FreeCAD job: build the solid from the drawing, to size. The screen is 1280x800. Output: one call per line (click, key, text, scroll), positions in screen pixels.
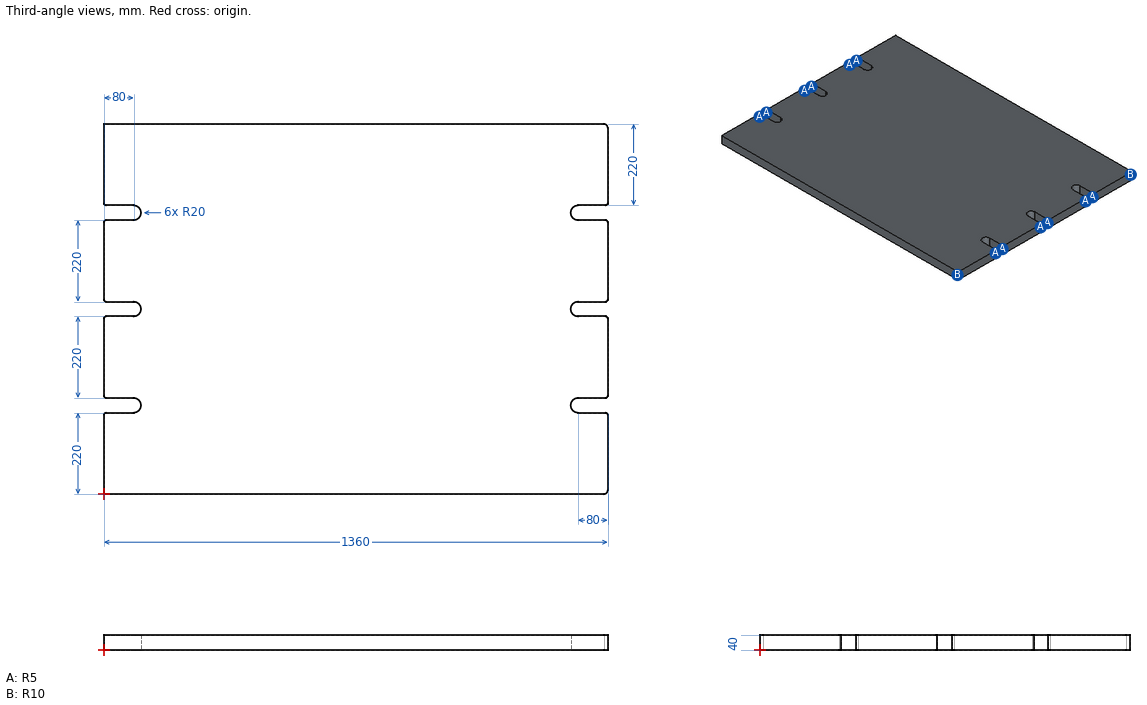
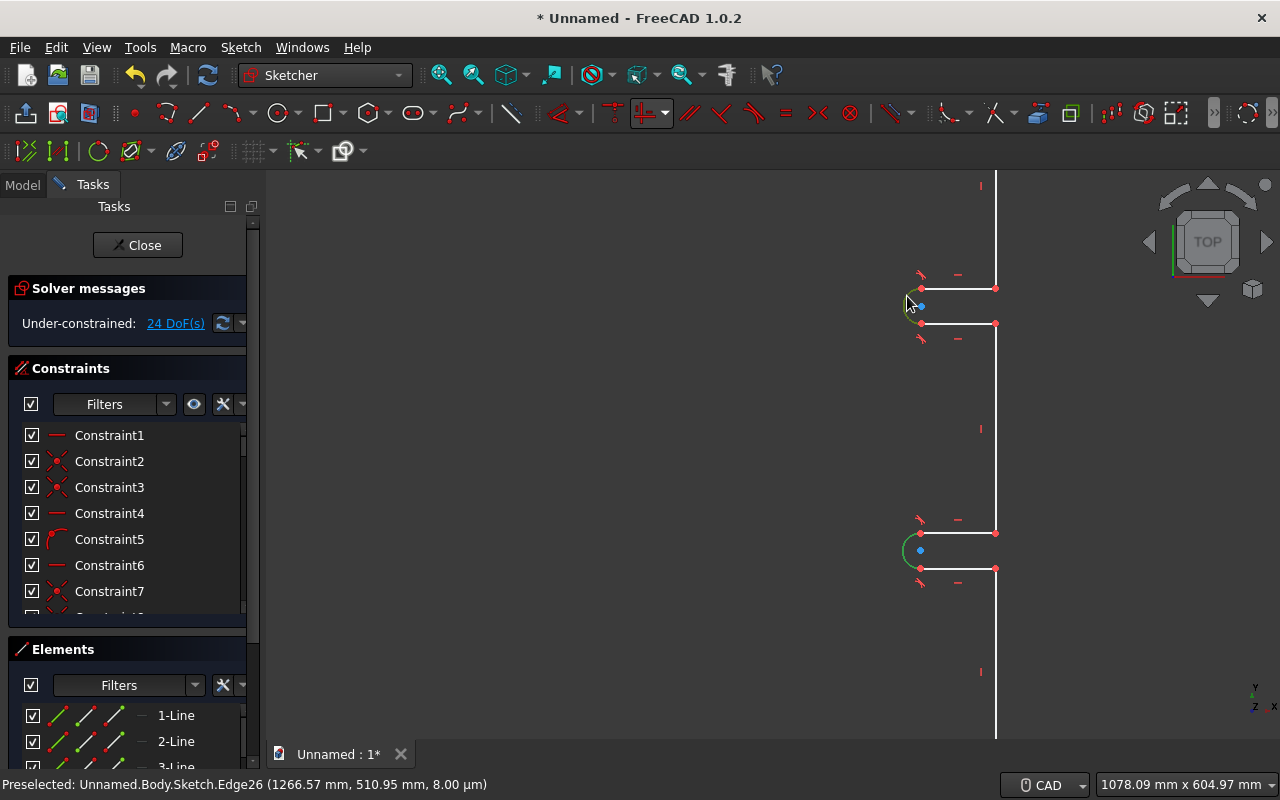
scroll(907, 542, down, 5)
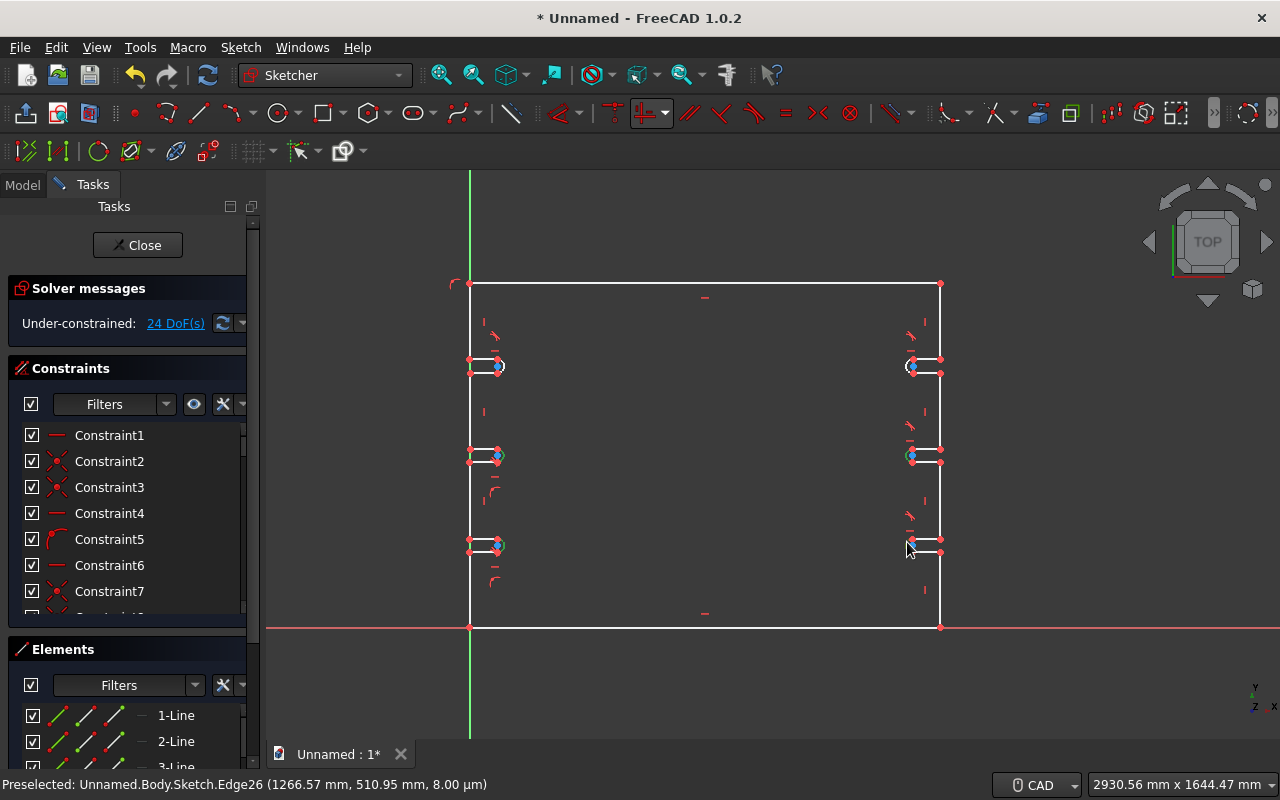
scroll(907, 362, up, 4)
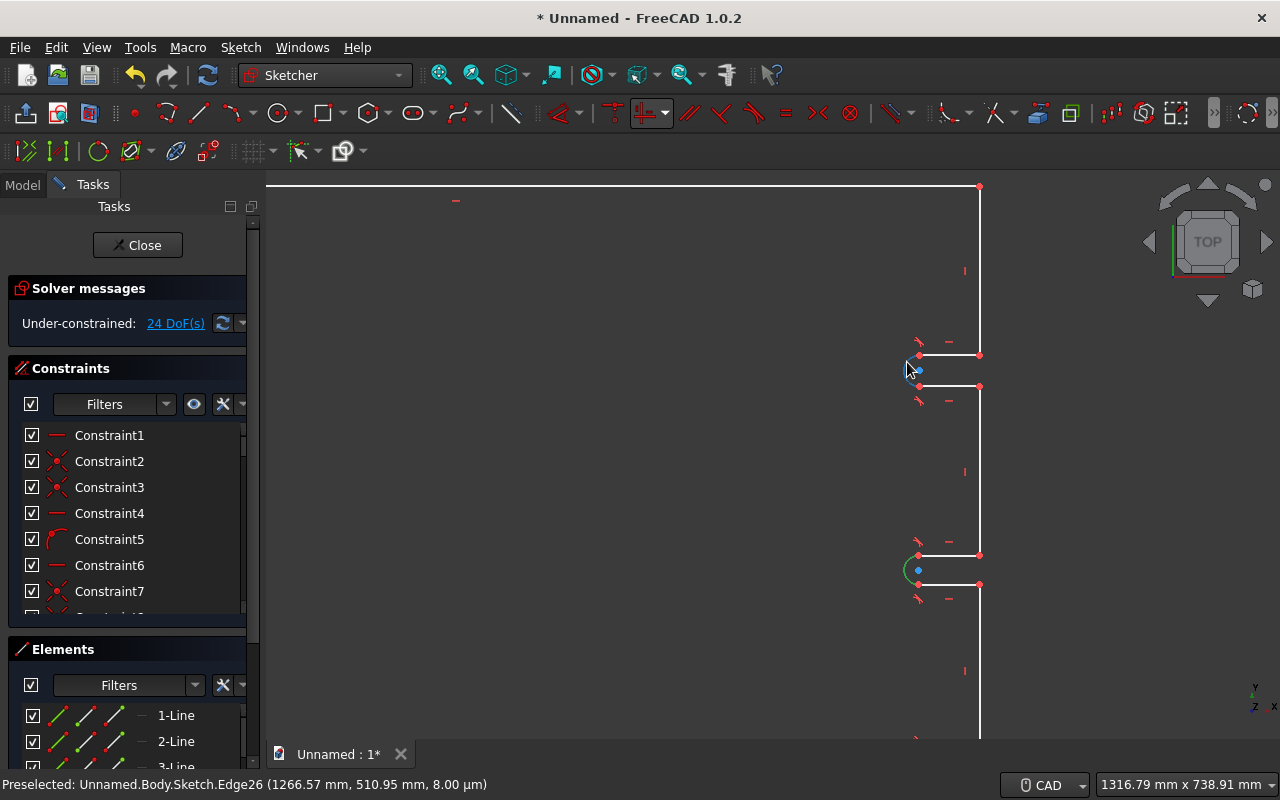
click(907, 362)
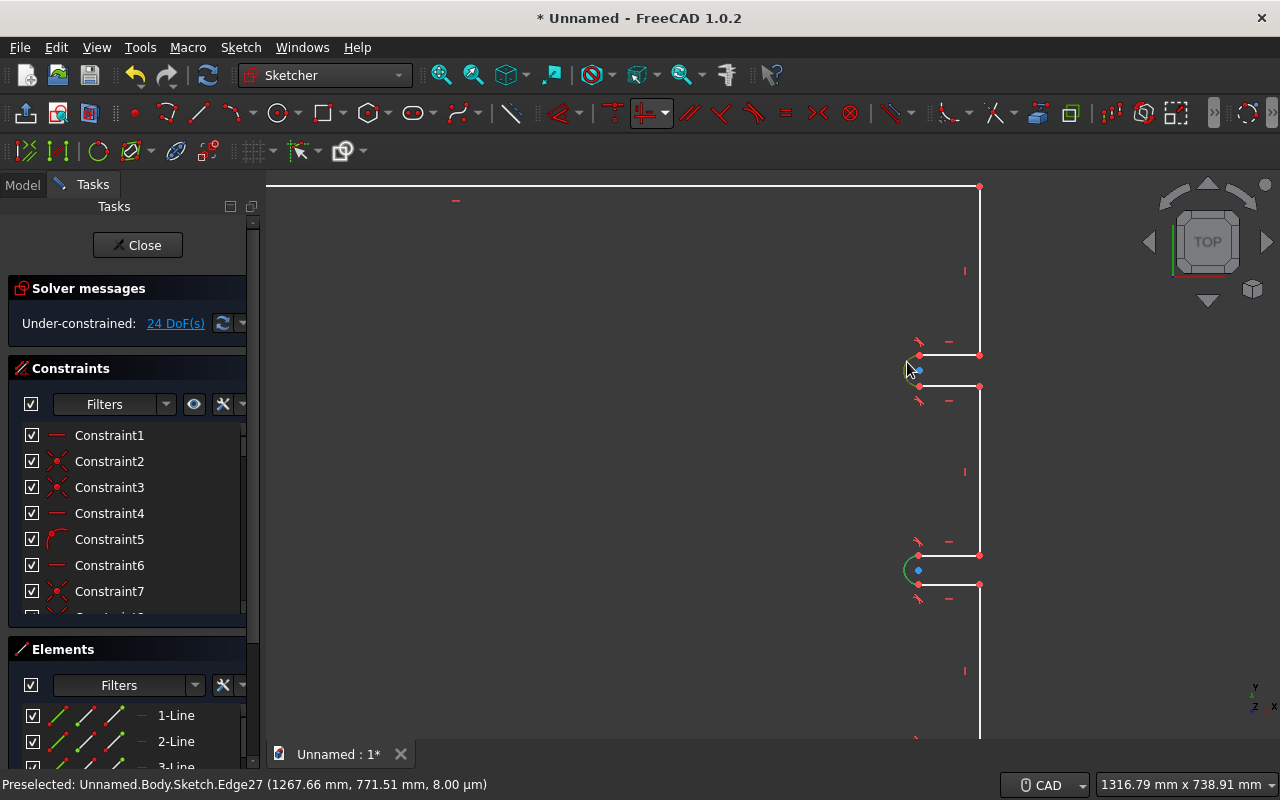
scroll(906, 362, down, 4)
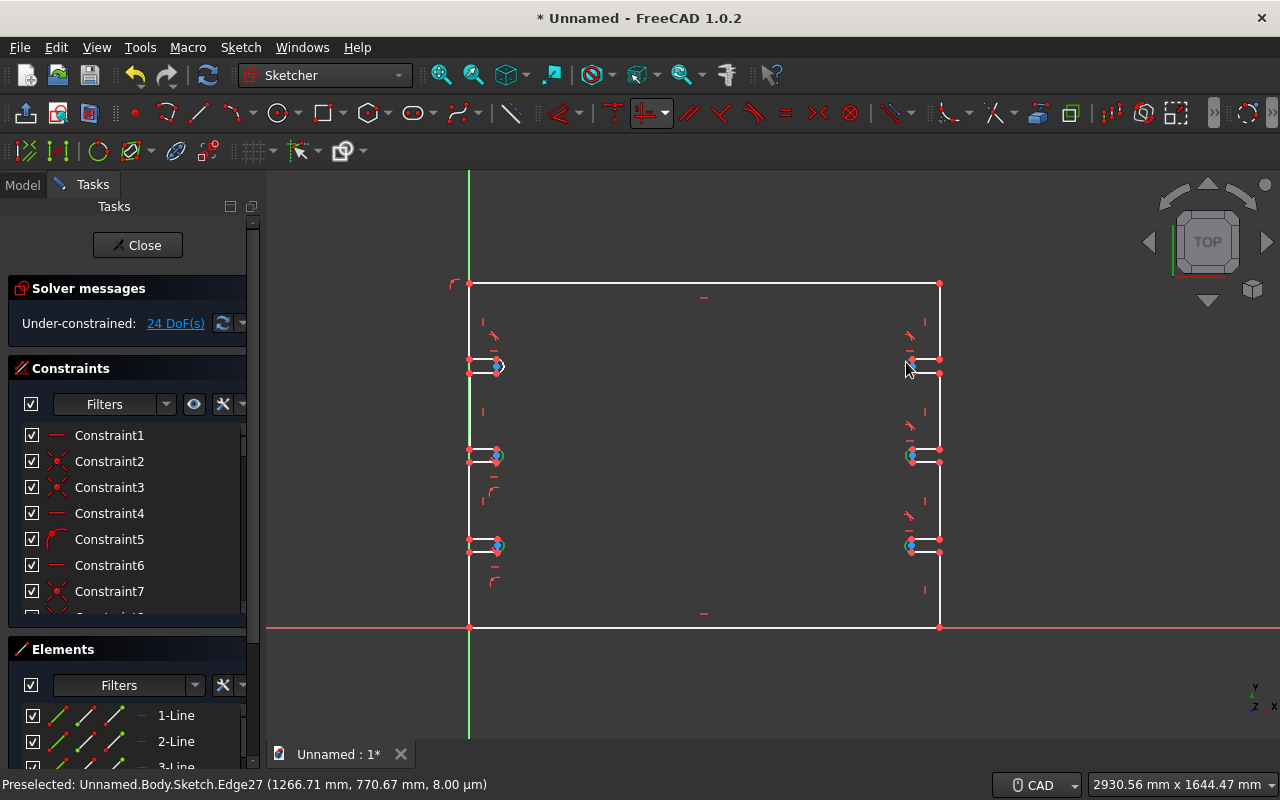
scroll(502, 370, up, 4)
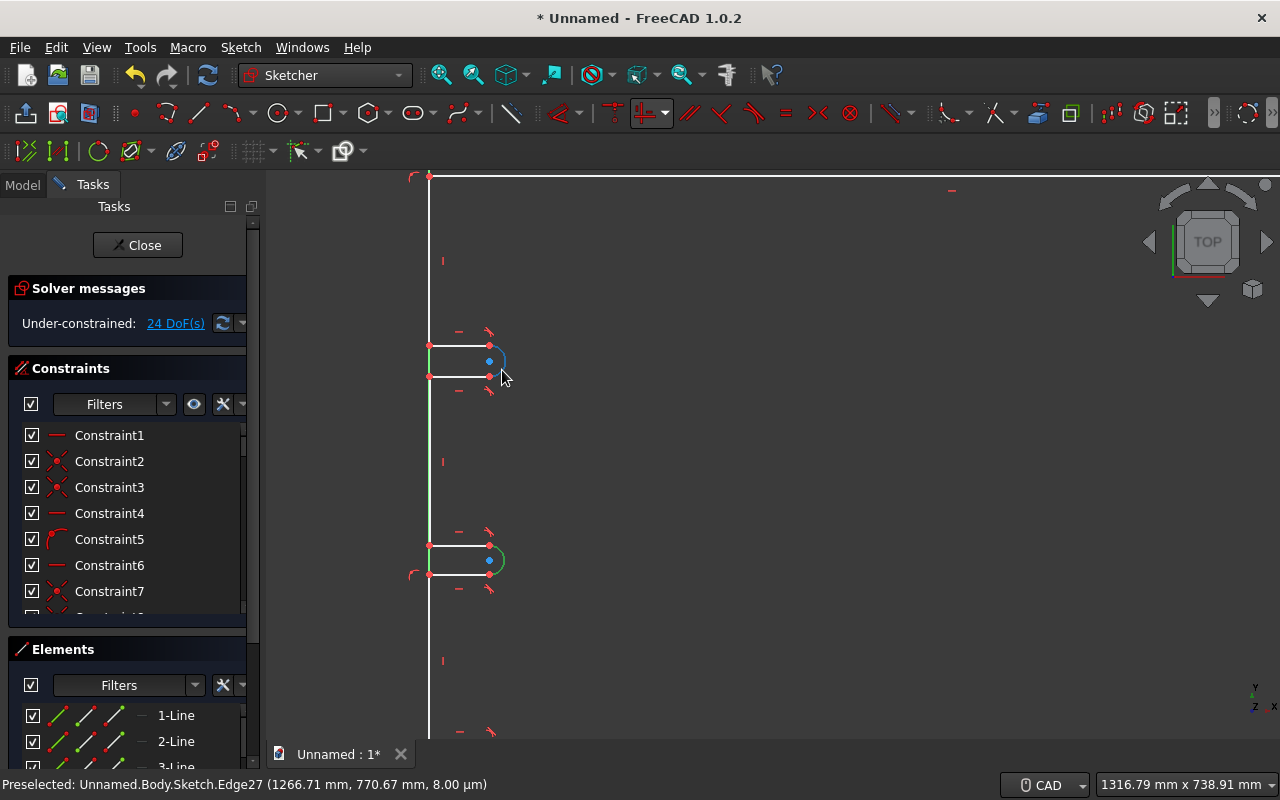
click(503, 370)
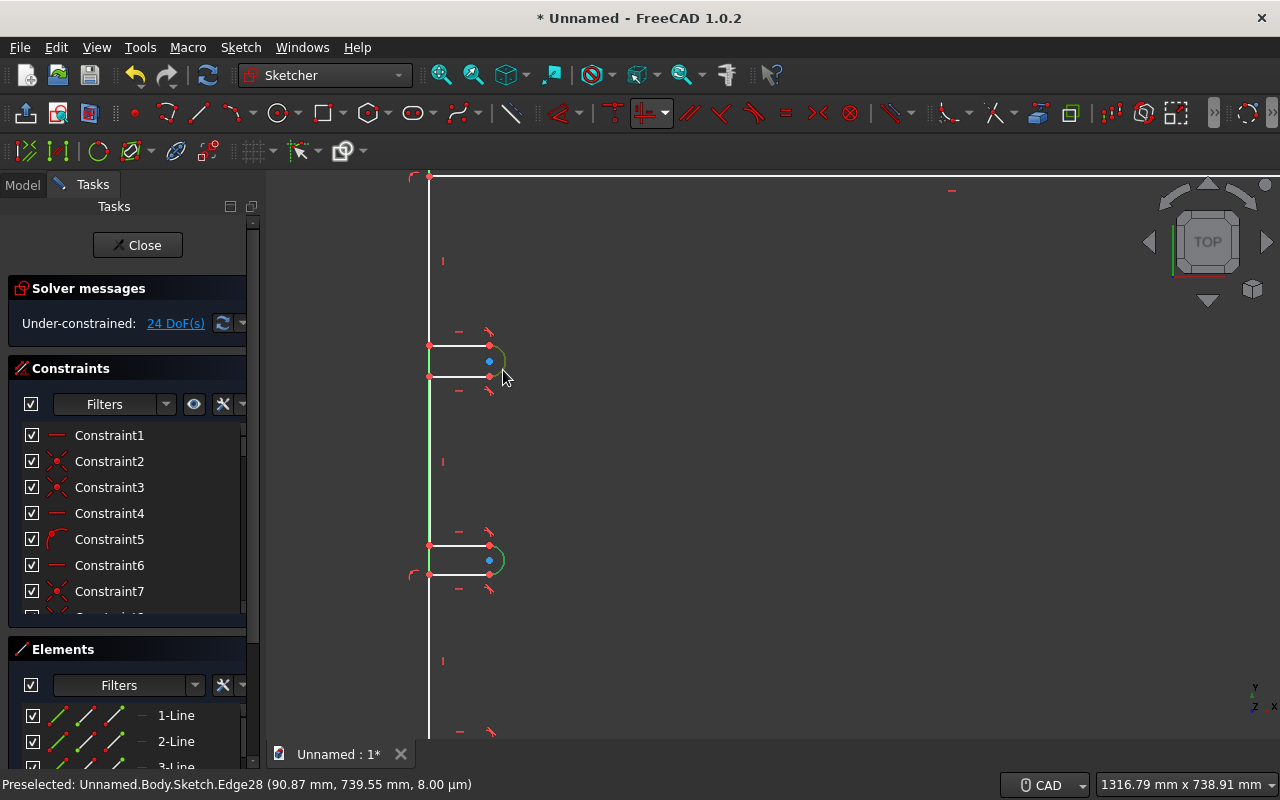
click(786, 114)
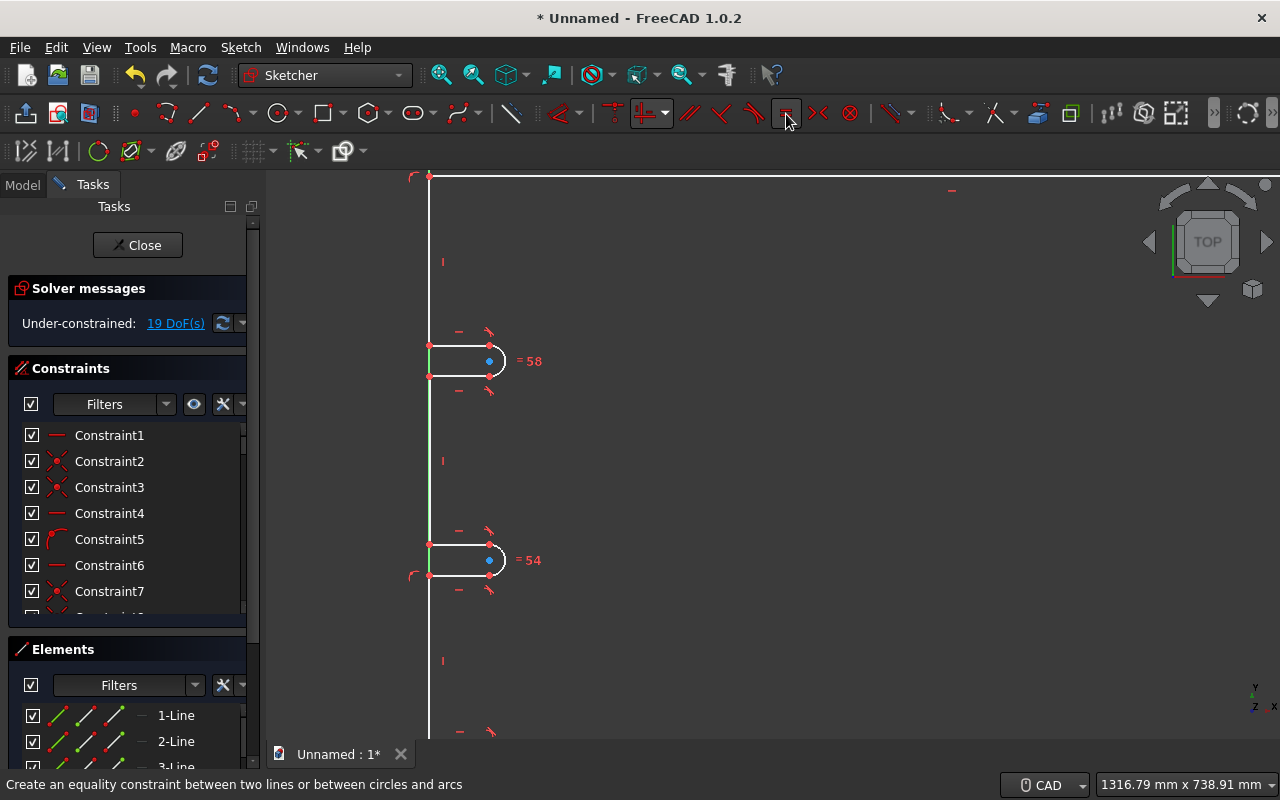
scroll(502, 569, up, 5)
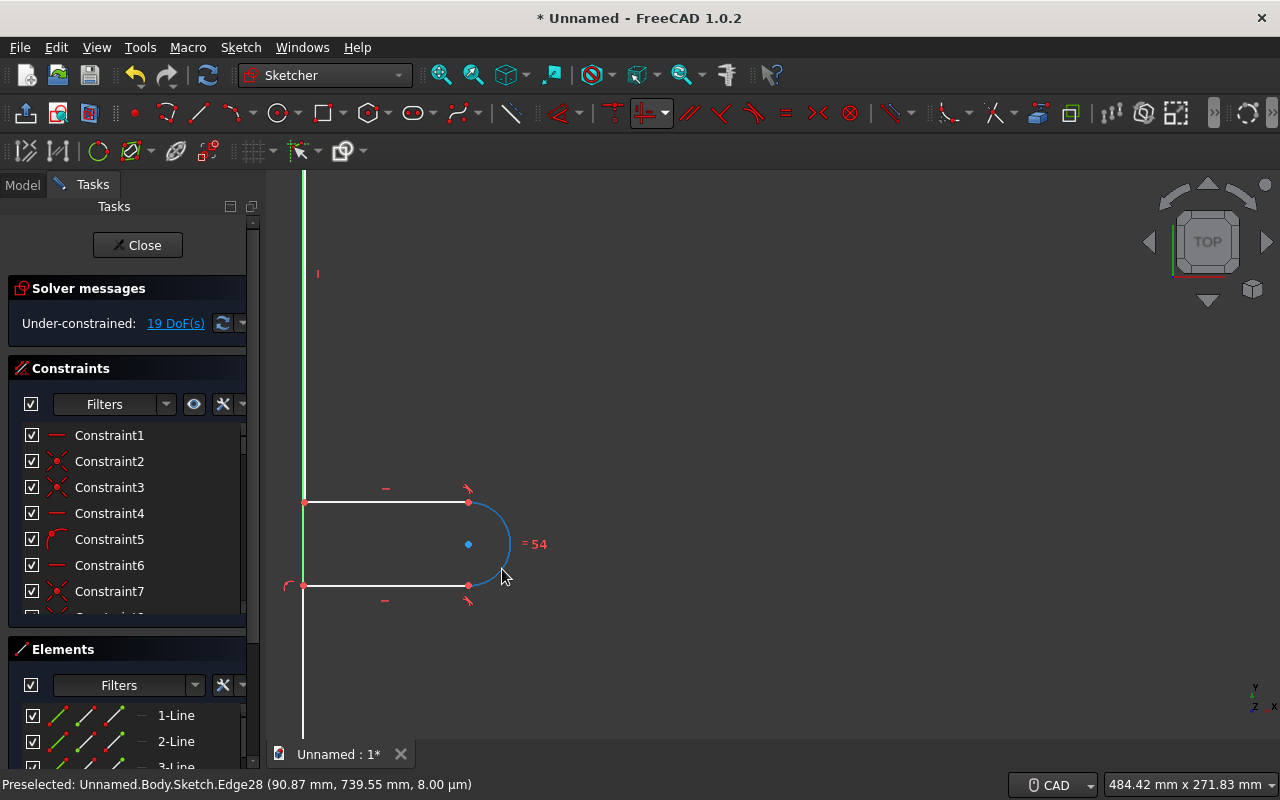
click(502, 569)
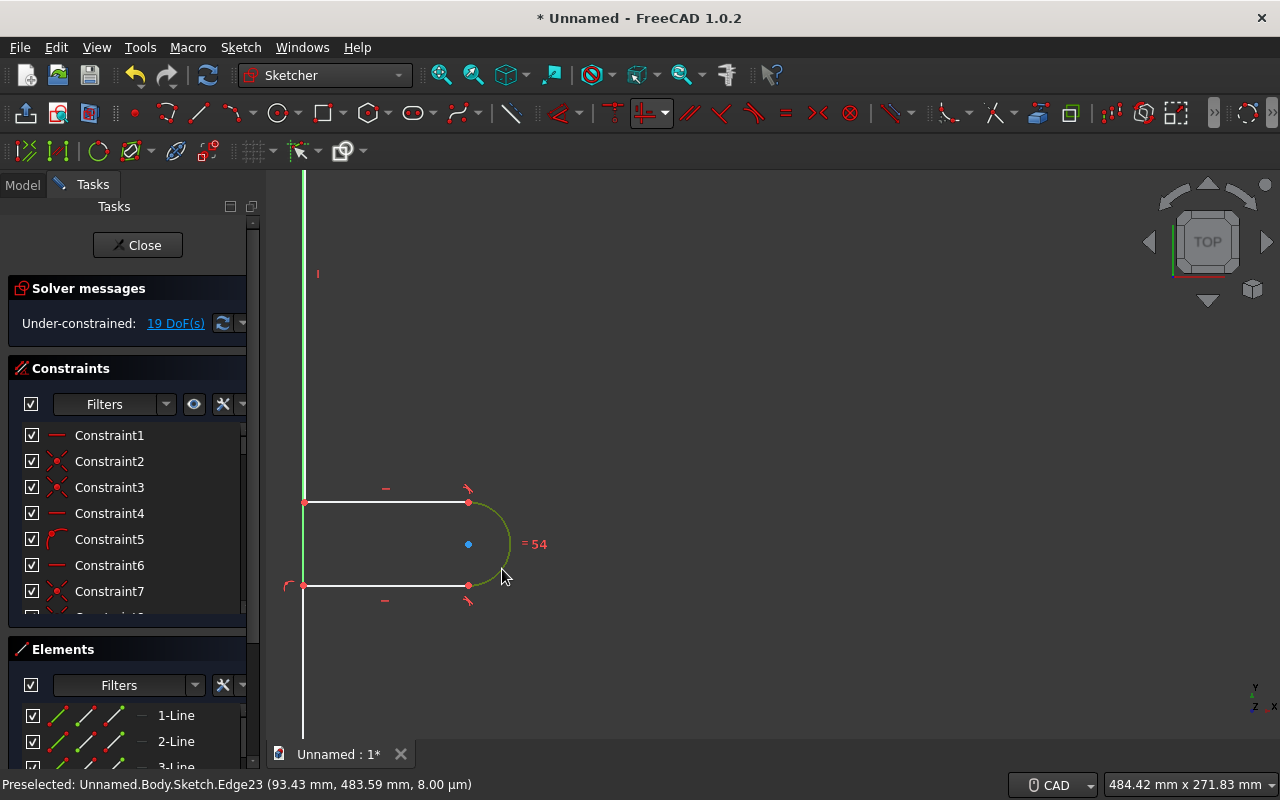
click(582, 114)